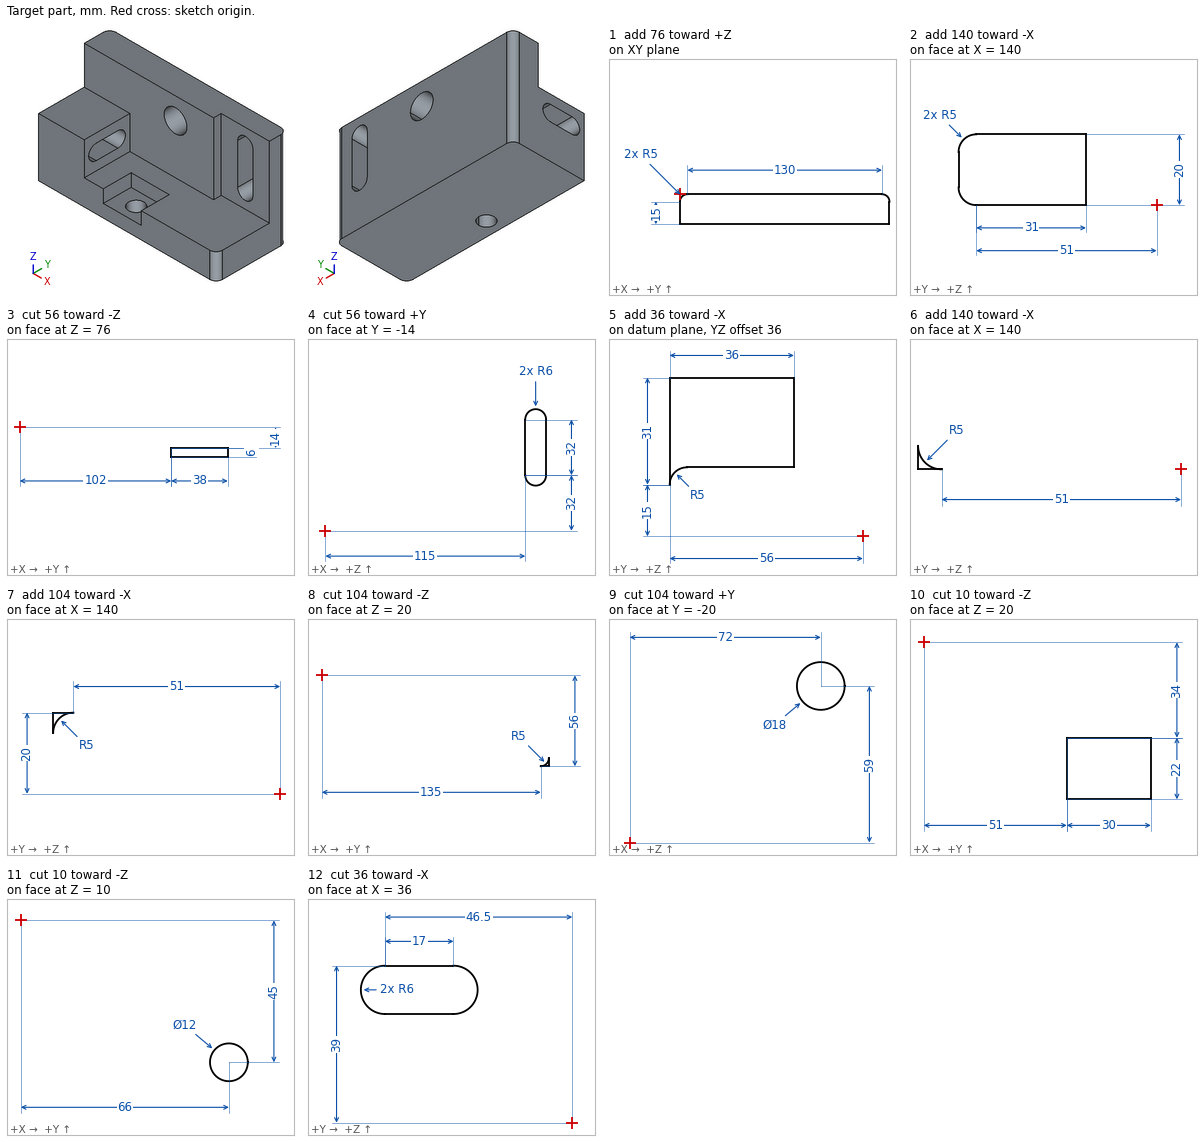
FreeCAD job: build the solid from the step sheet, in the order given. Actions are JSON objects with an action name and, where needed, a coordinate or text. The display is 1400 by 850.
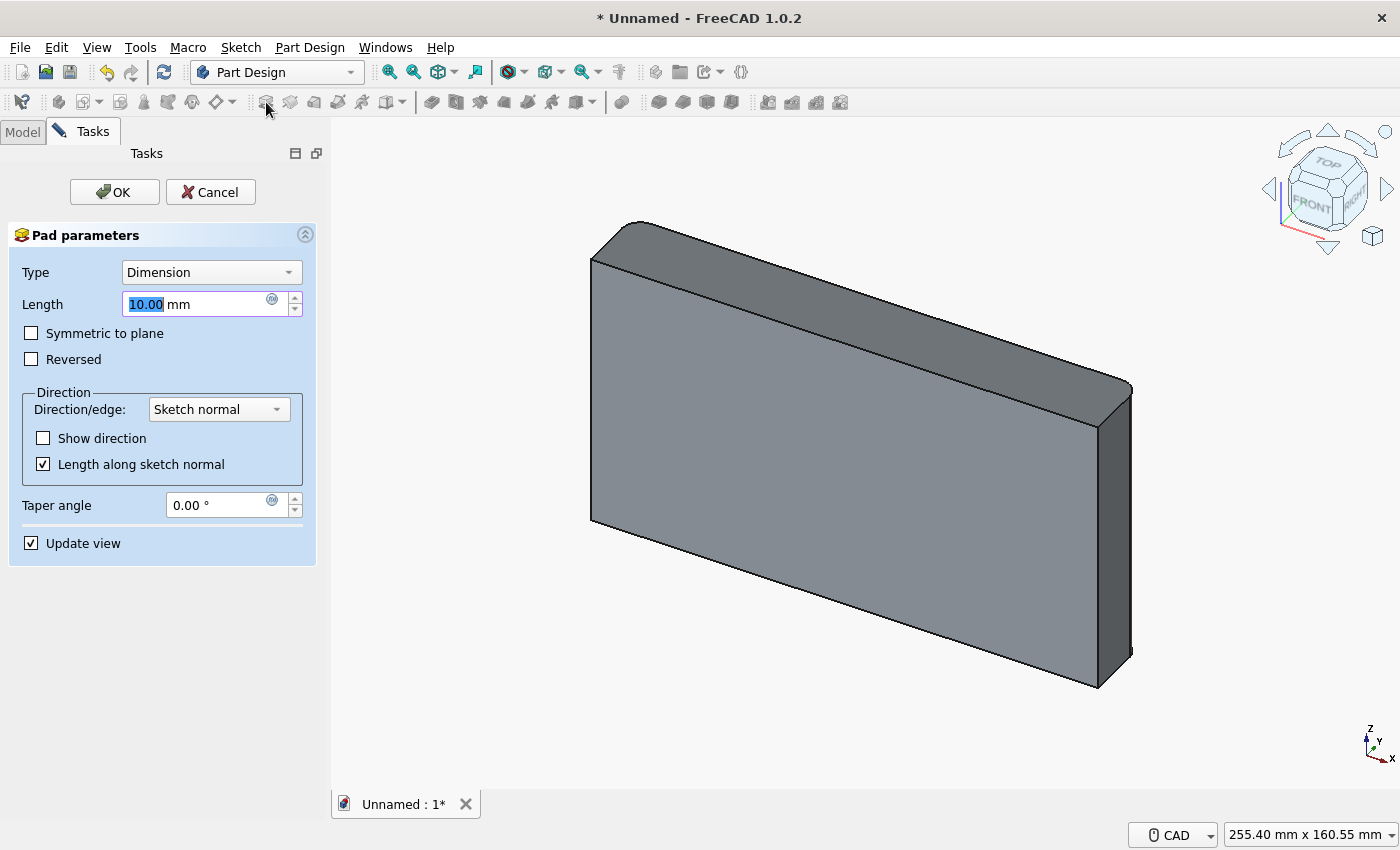
{"action": "type", "text": "140"}
{"action": "key", "text": "Tab"}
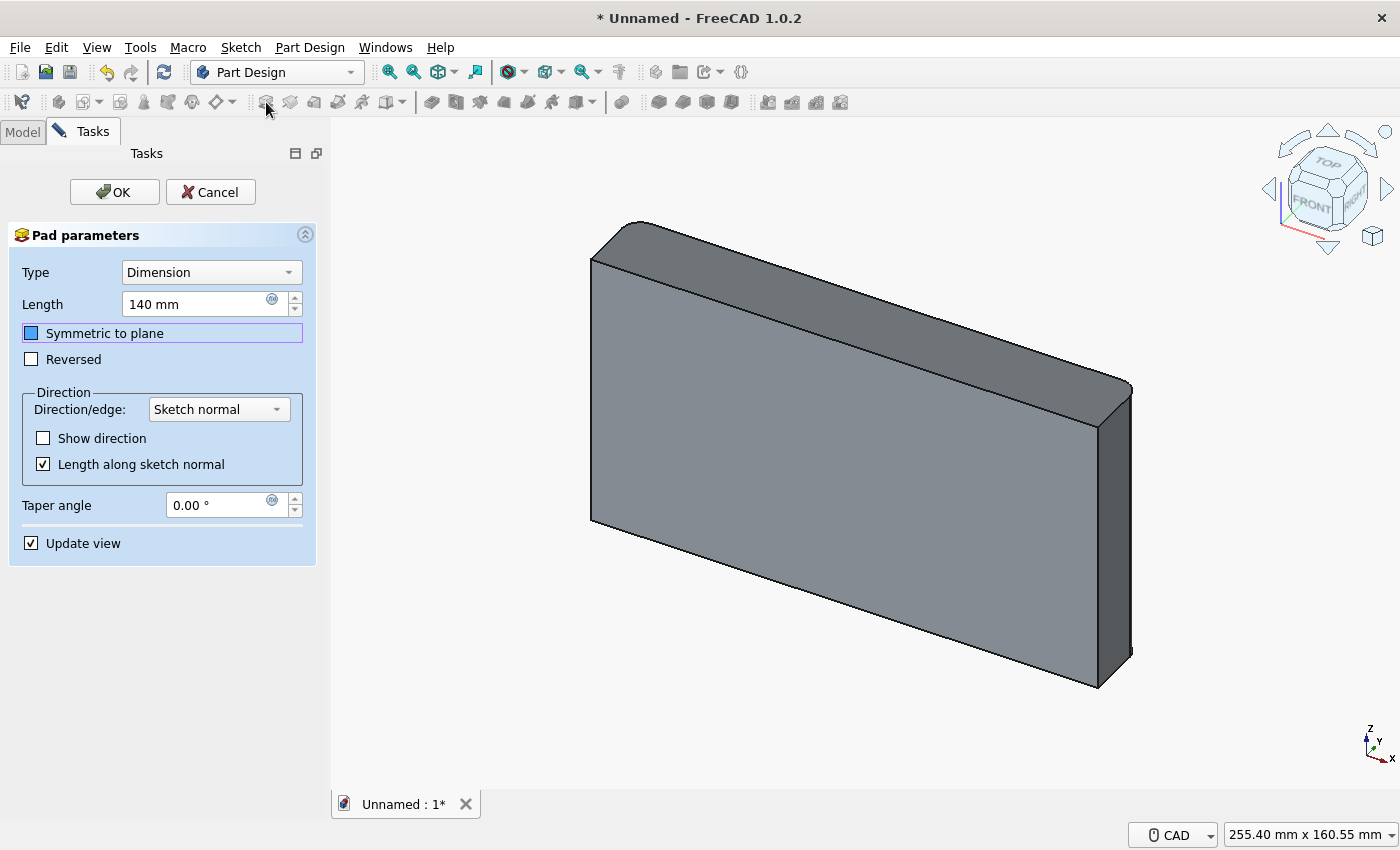
{"action": "left_click", "coordinate": [30, 359]}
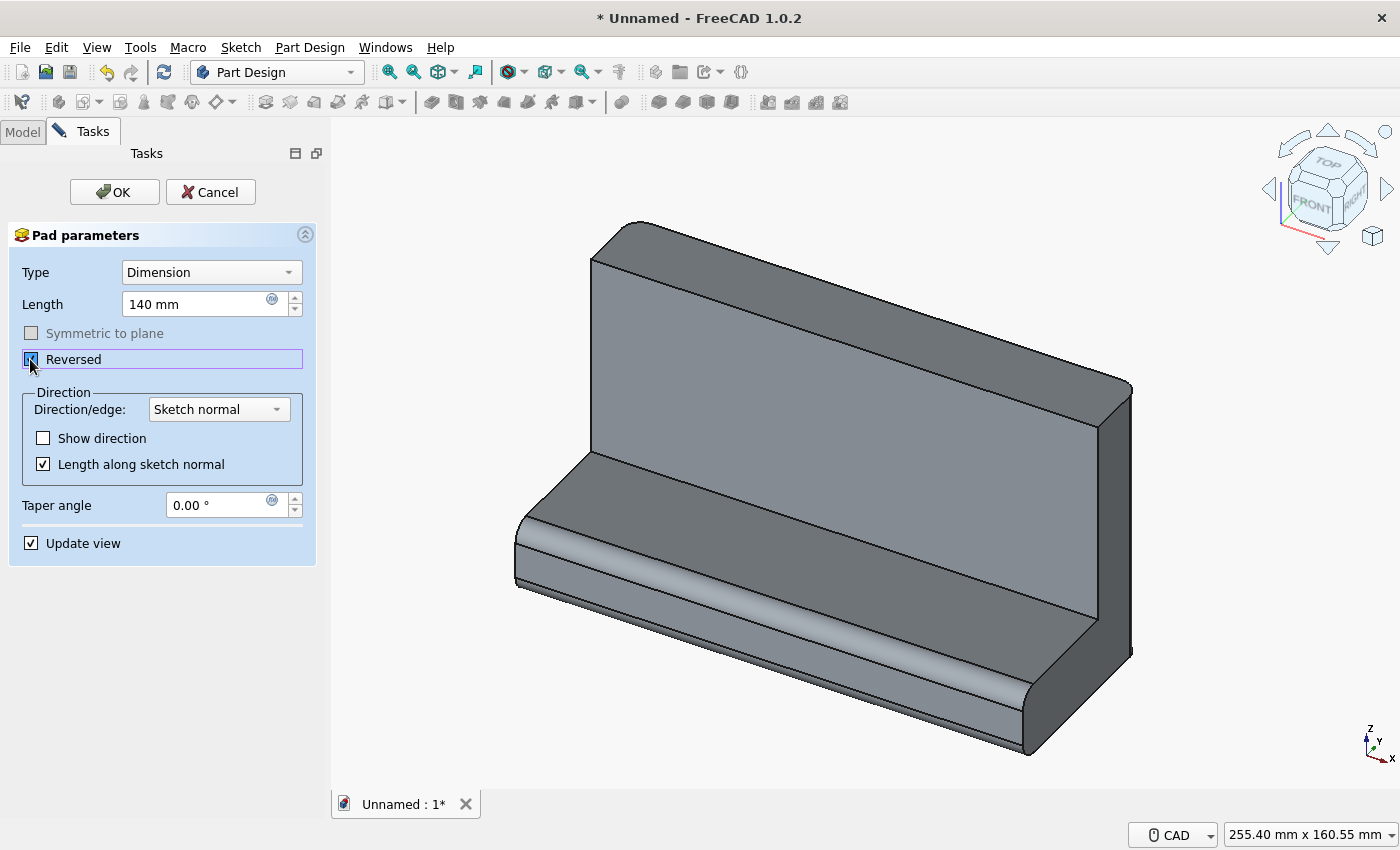
{"action": "left_click", "coordinate": [115, 192]}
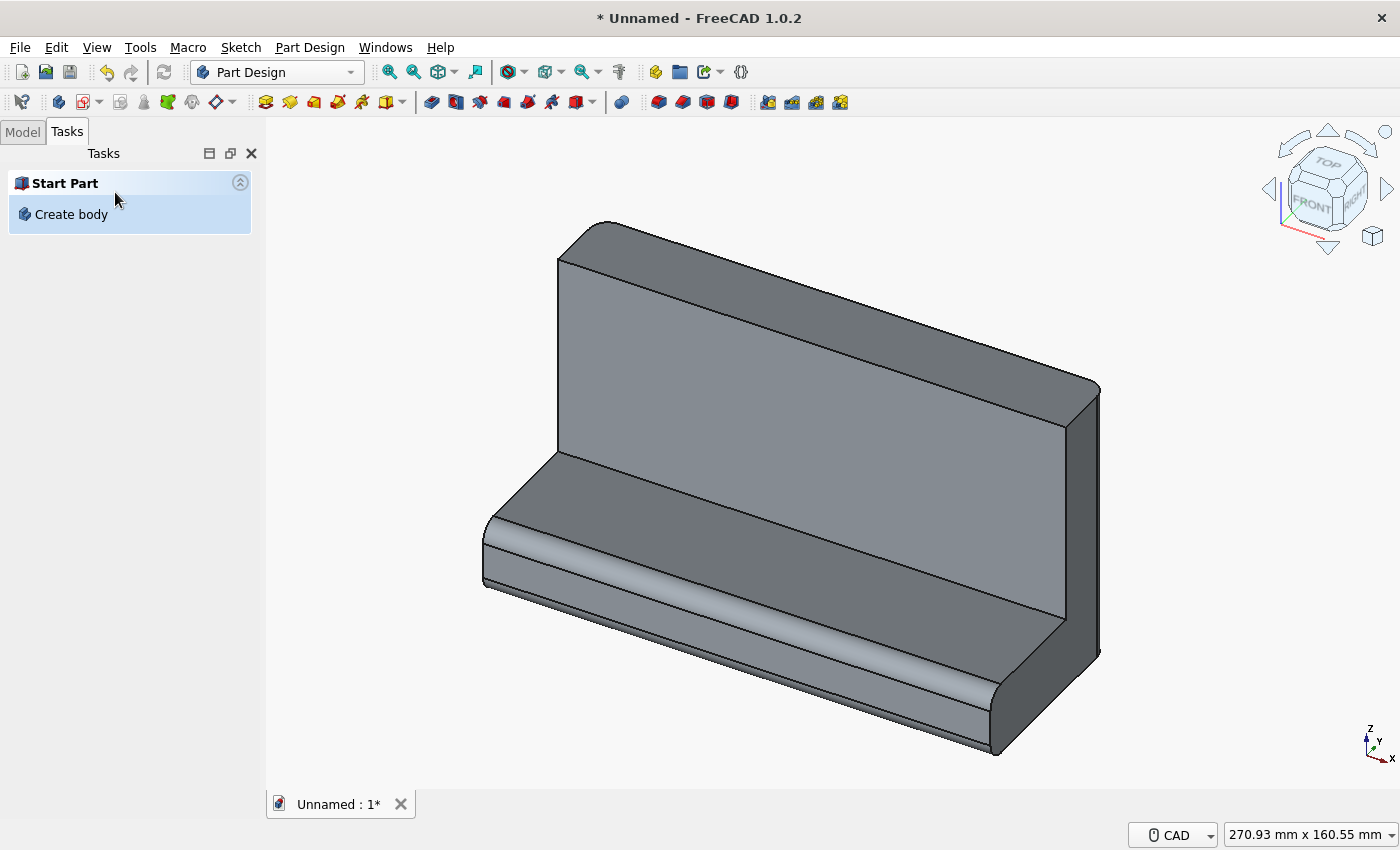
{"action": "left_click", "coordinate": [1050, 394]}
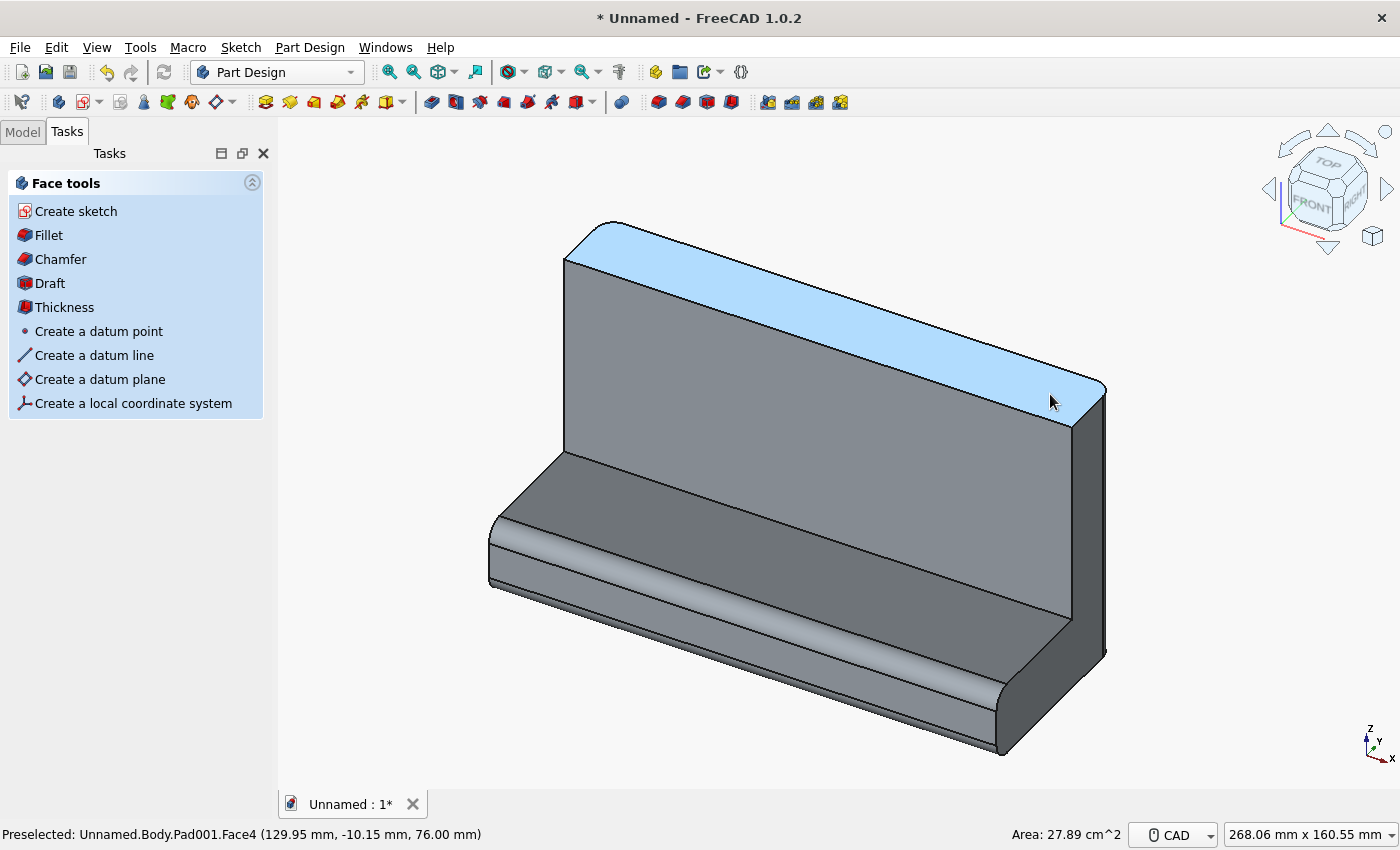
{"action": "left_click", "coordinate": [84, 102]}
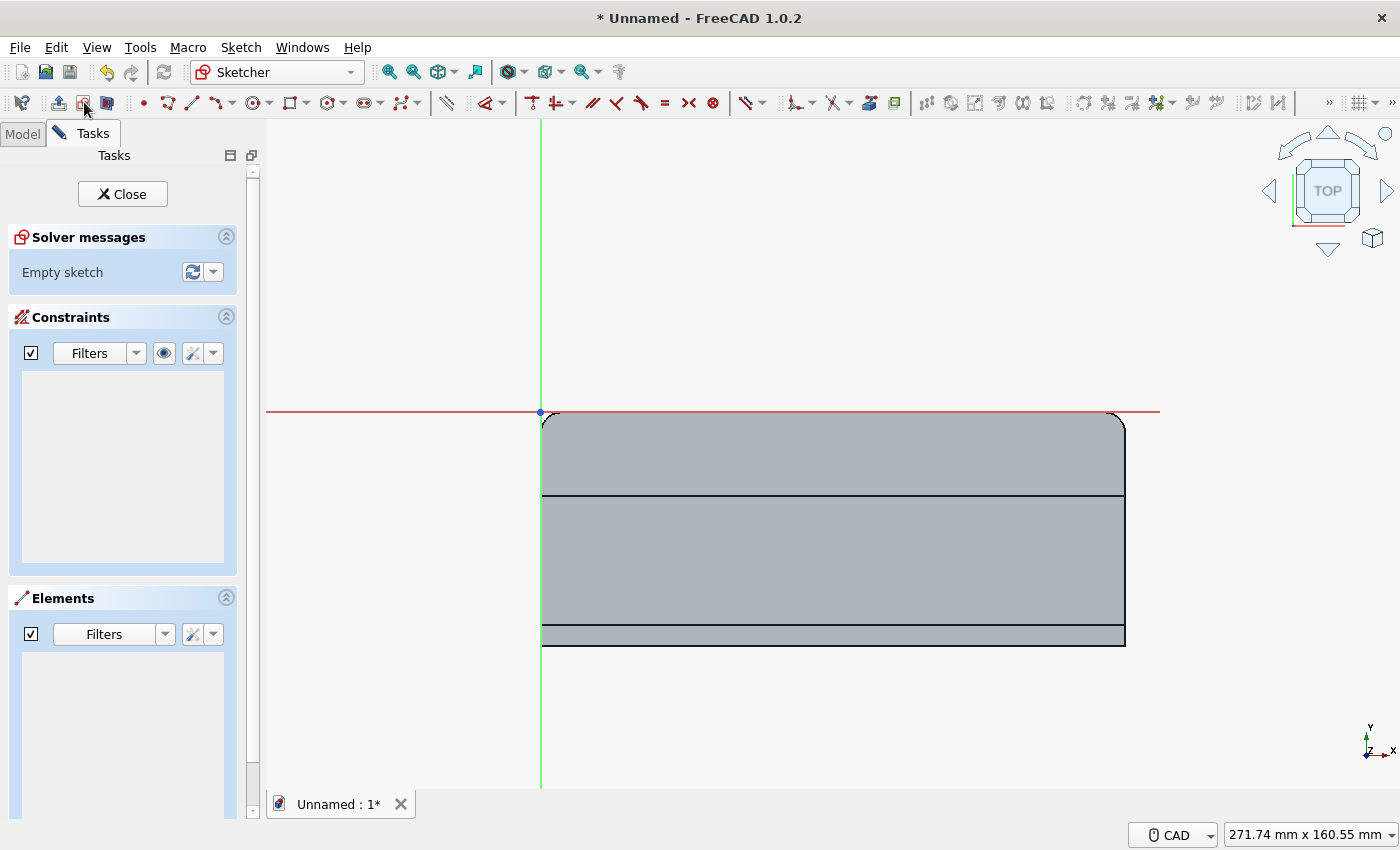
{"action": "scroll", "coordinate": [1138, 493], "scroll_direction": "up", "scroll_amount": 7}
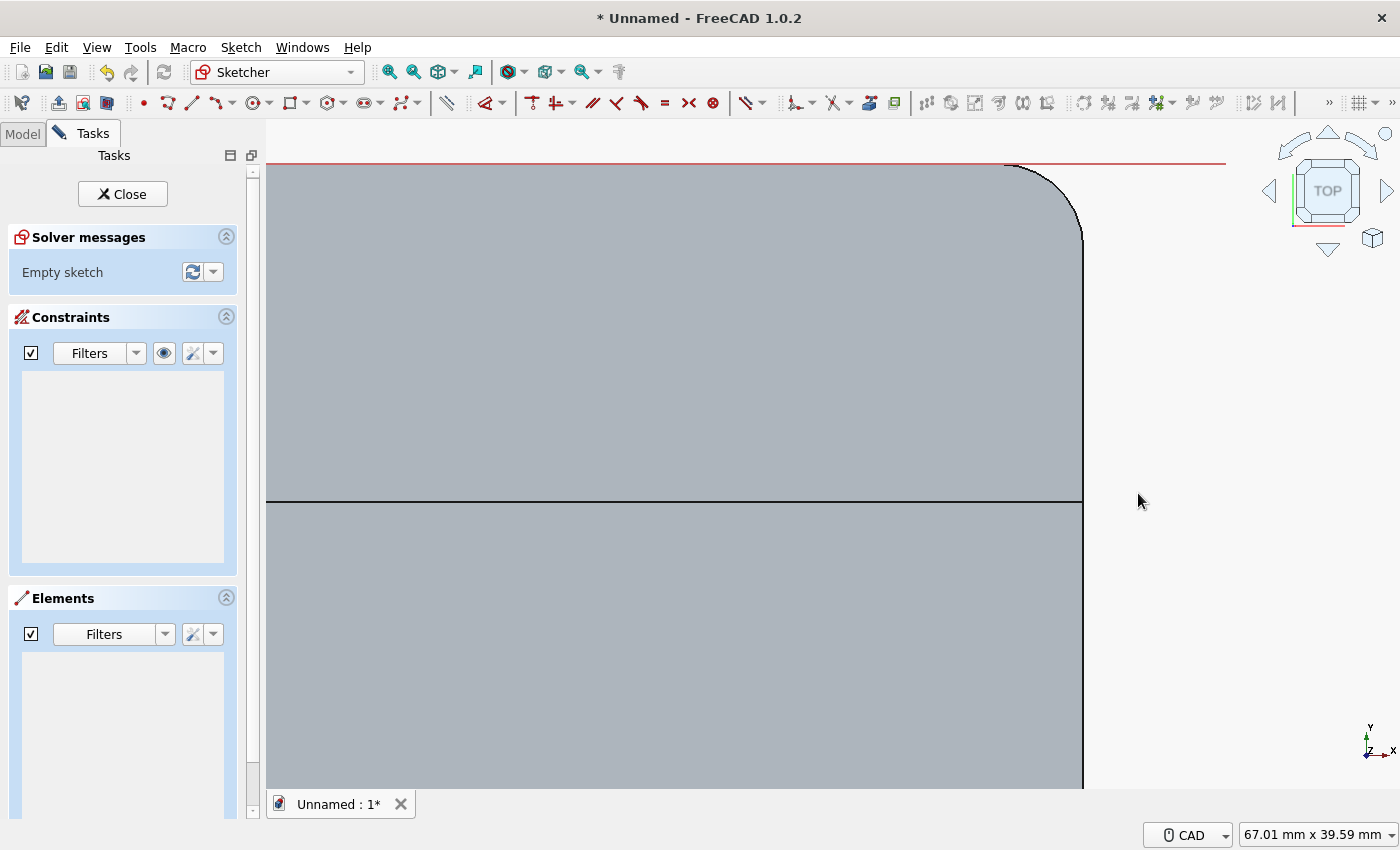
{"action": "left_click", "coordinate": [290, 104]}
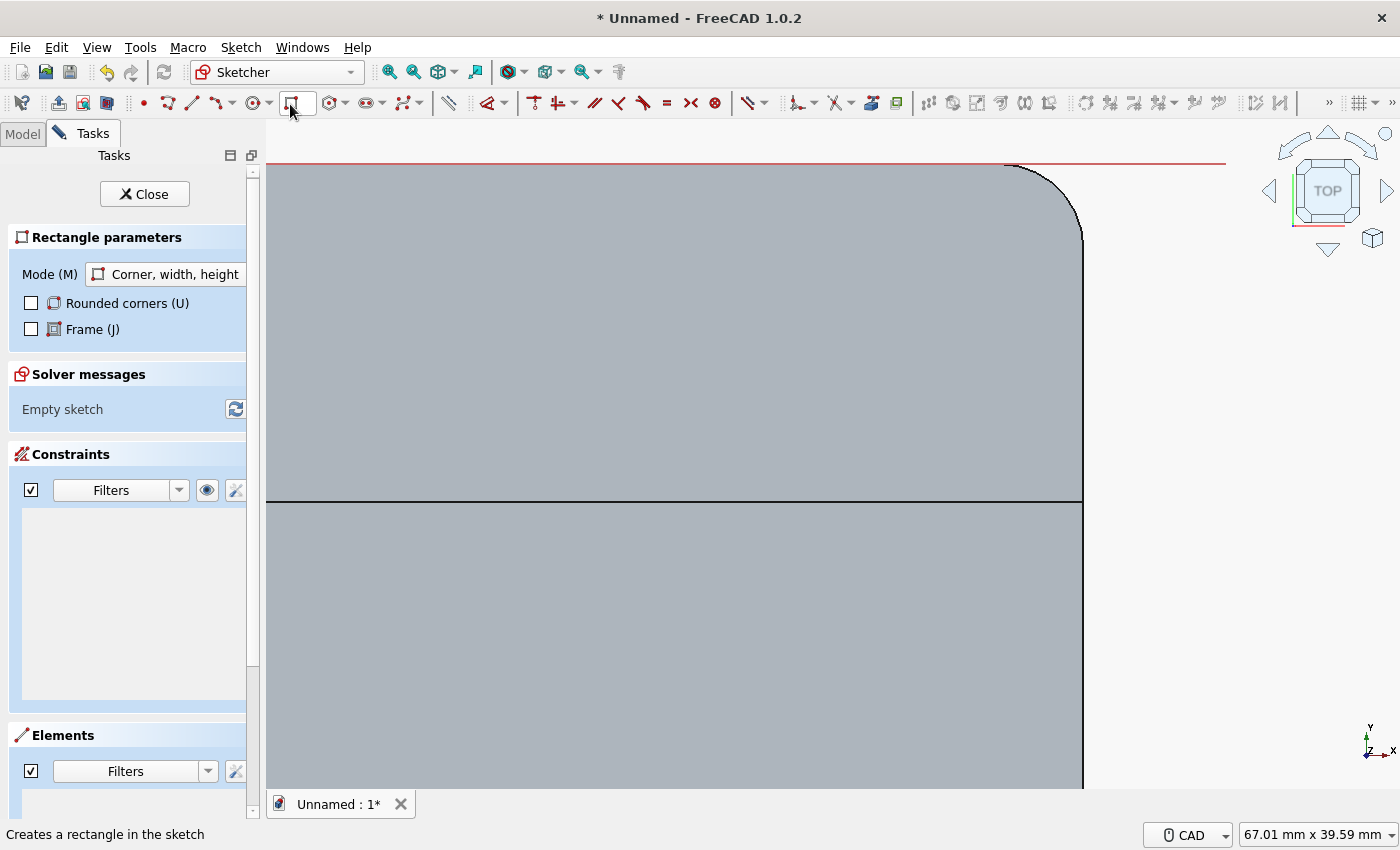
{"action": "left_click", "coordinate": [440, 401]}
{"action": "left_click", "coordinate": [1083, 502]}
{"action": "key", "text": "Escape"}